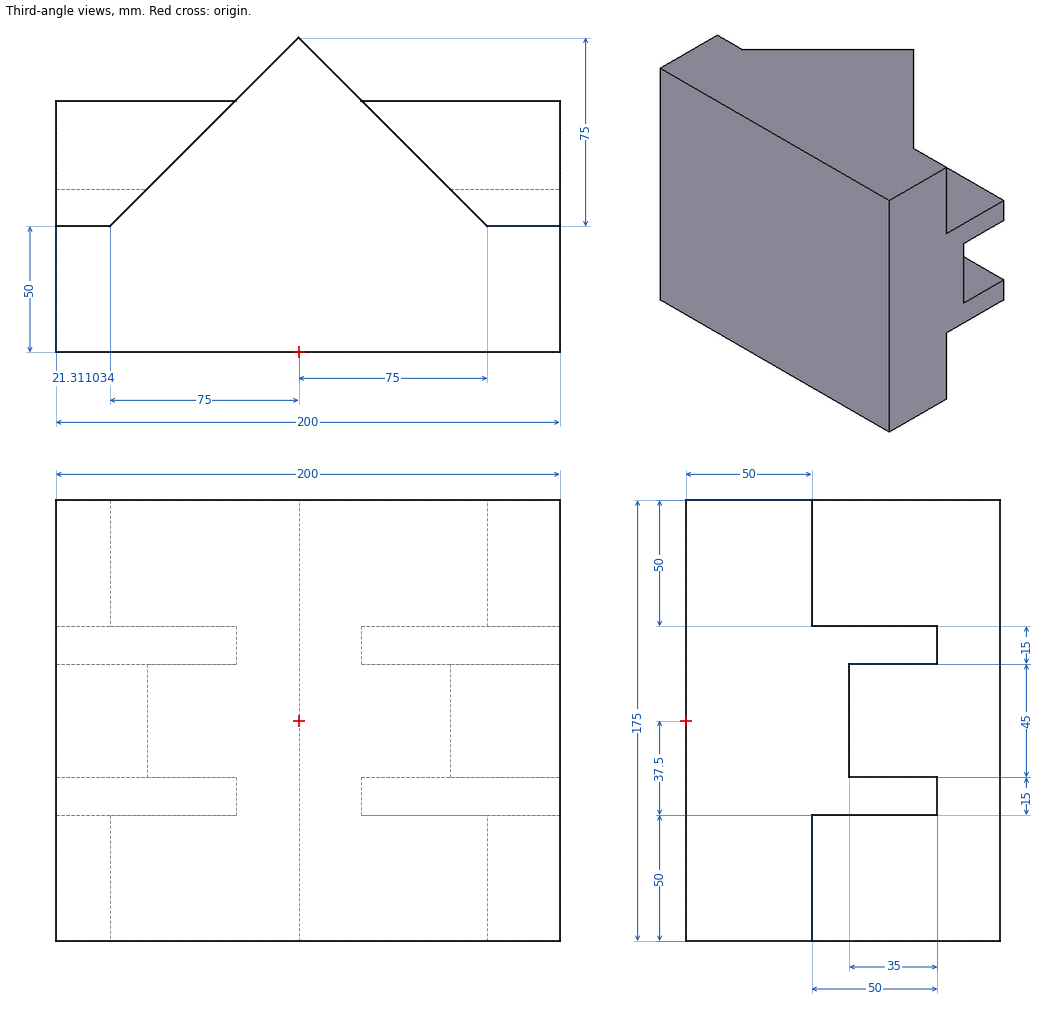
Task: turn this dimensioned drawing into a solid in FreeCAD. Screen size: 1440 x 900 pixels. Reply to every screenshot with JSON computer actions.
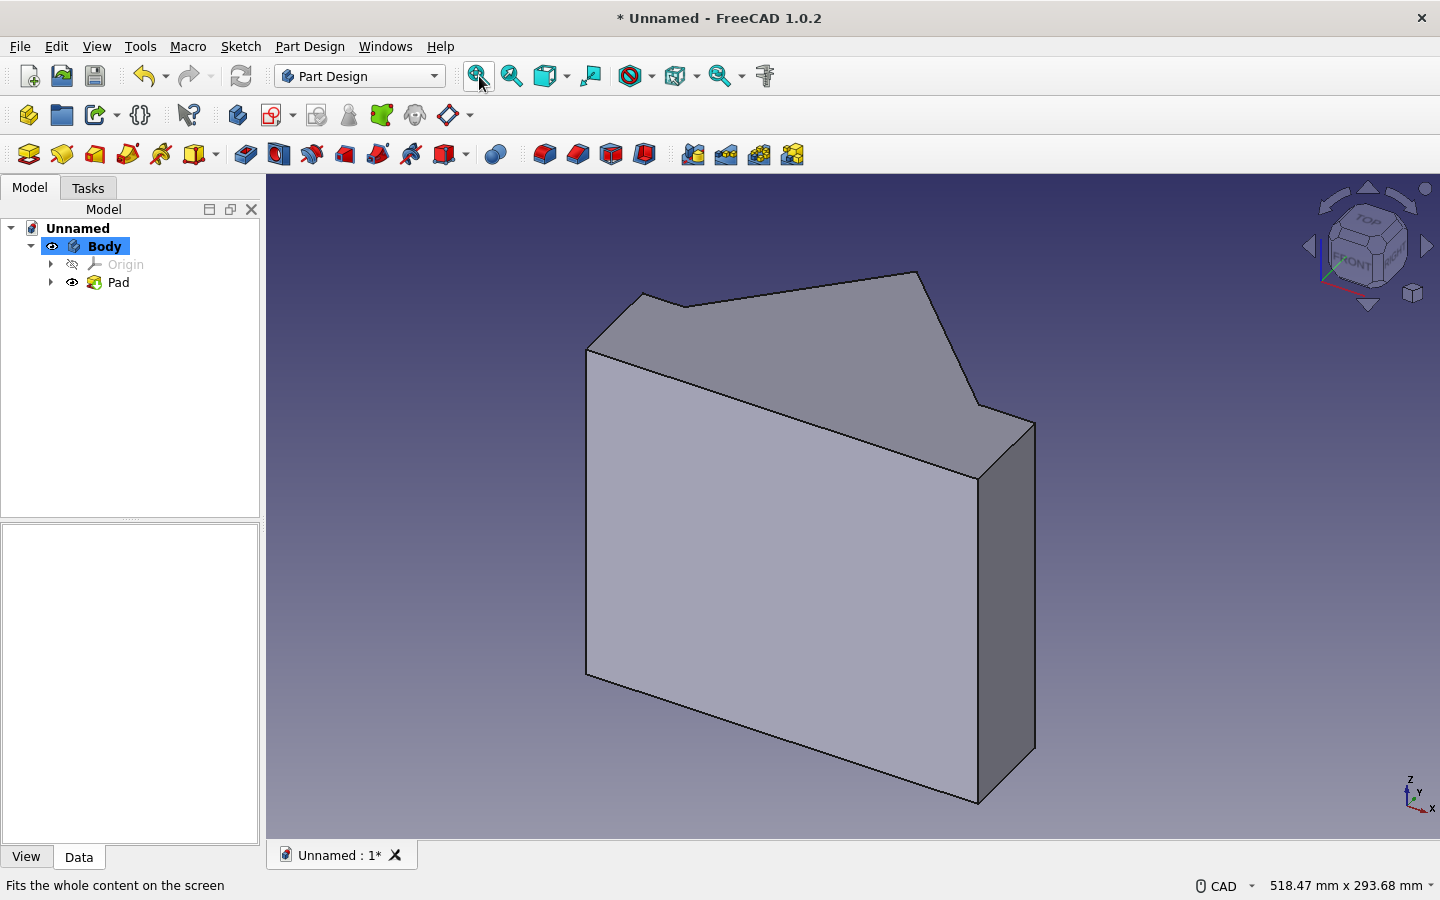
{"action": "key", "text": "6"}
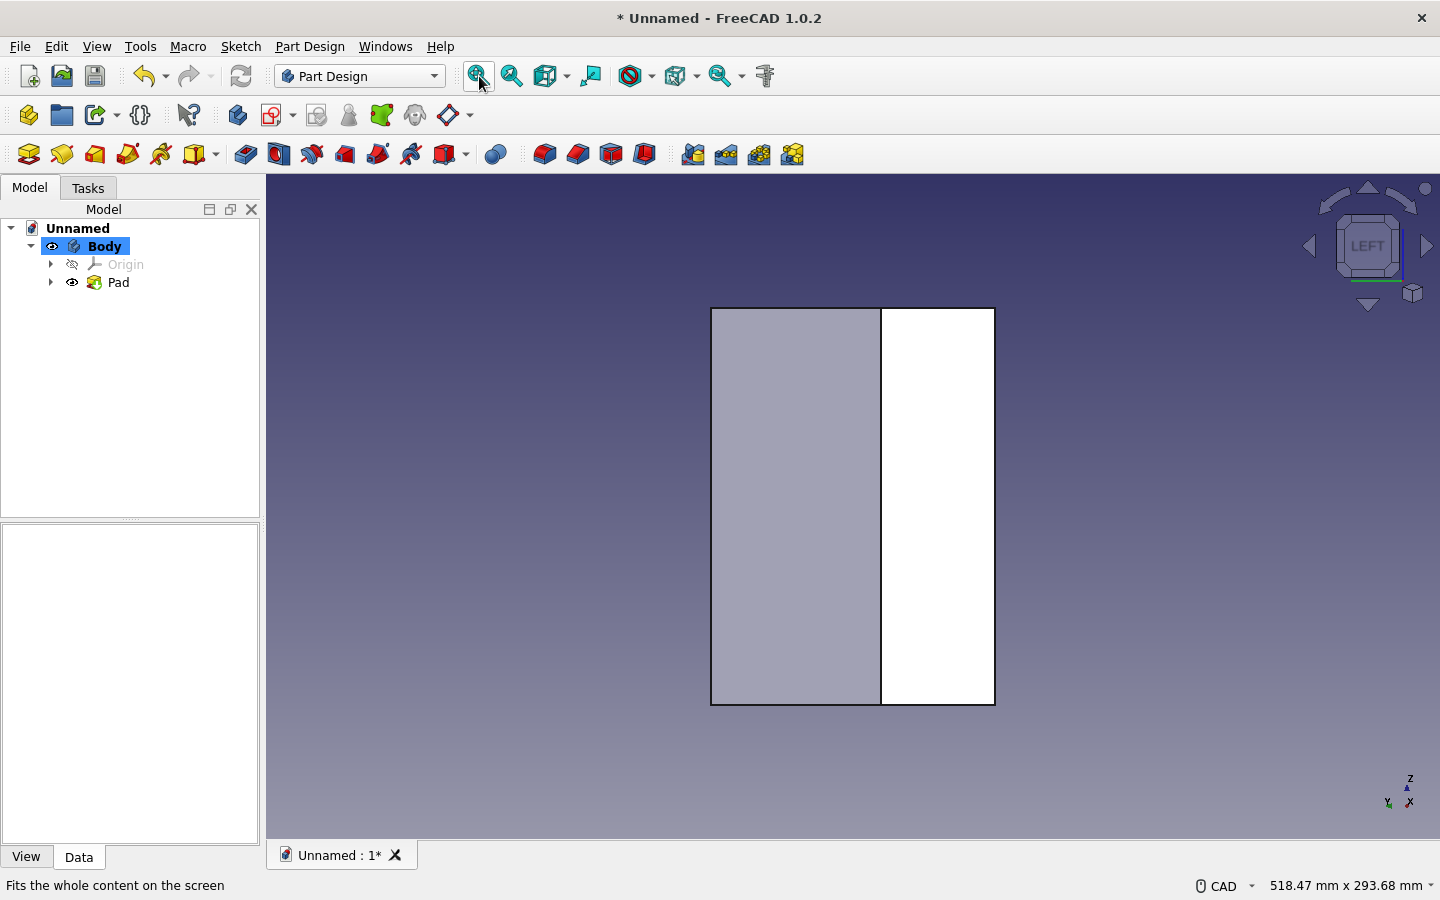
{"action": "left_click", "coordinate": [938, 392]}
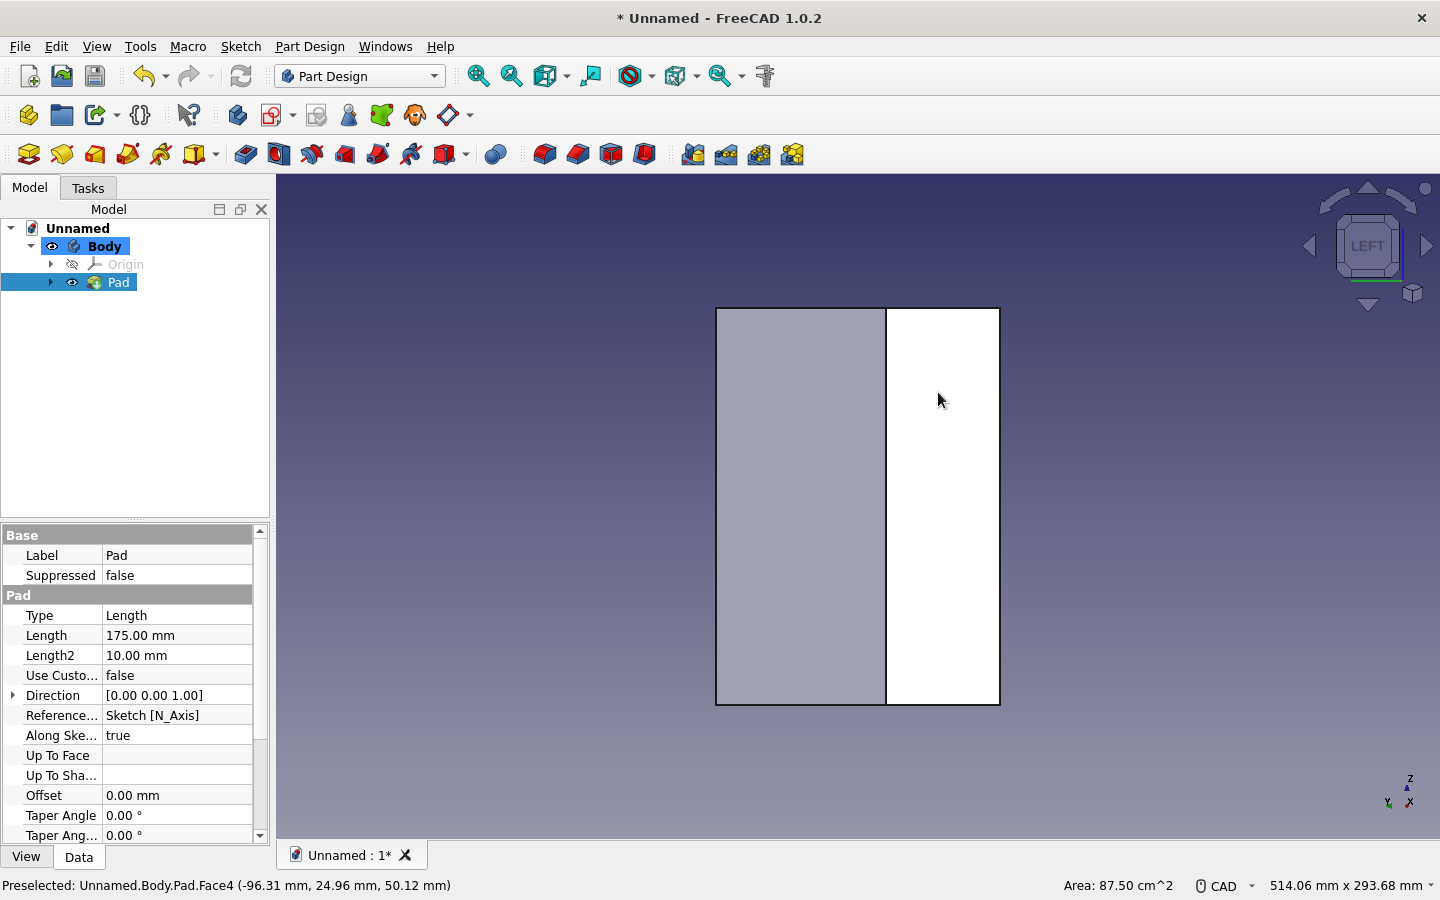
{"action": "left_click", "coordinate": [270, 116]}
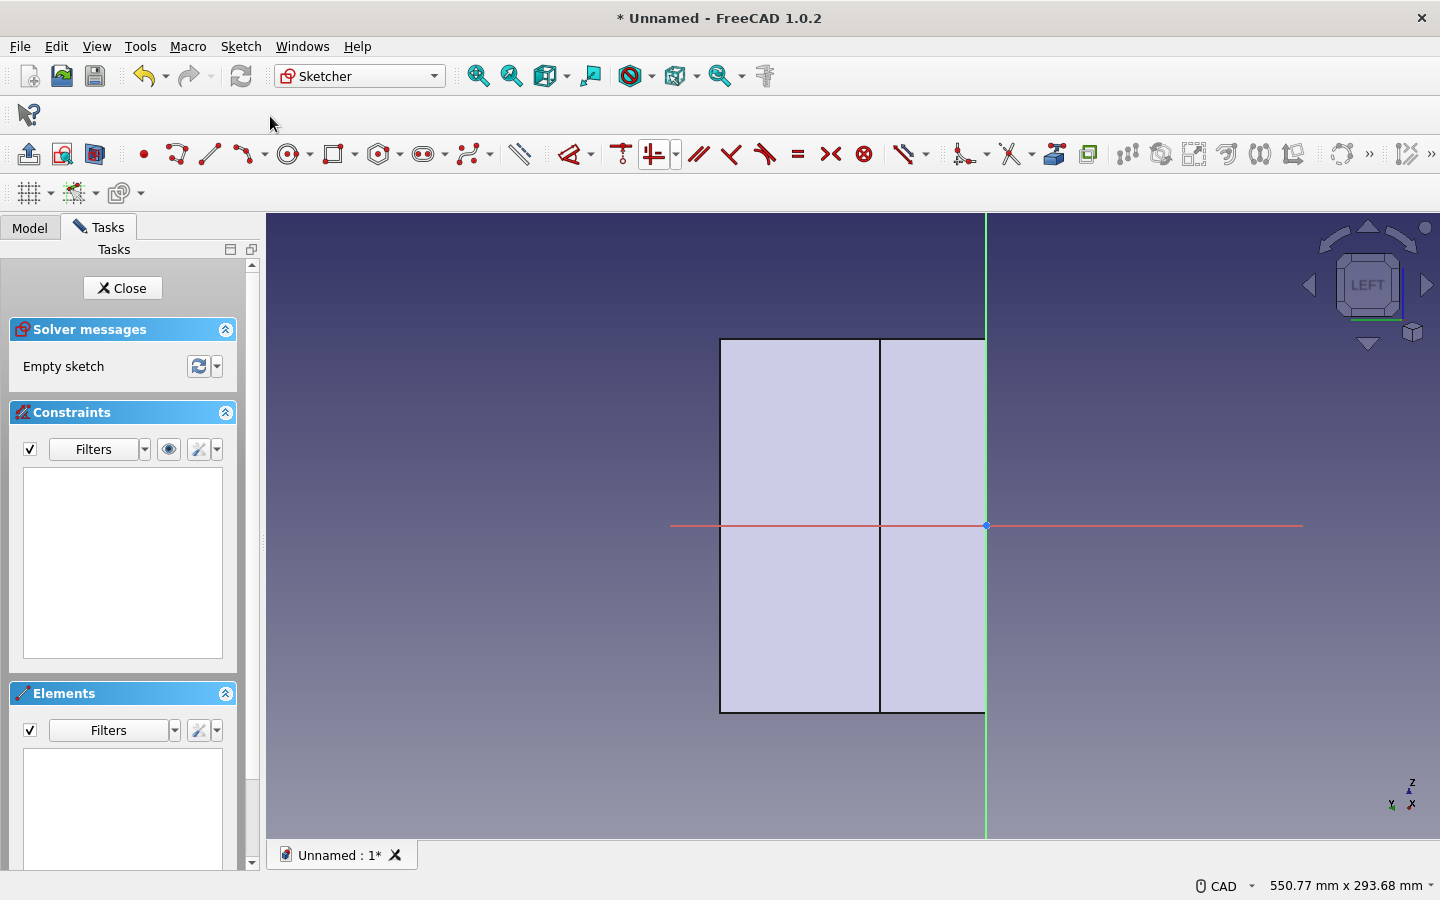
{"action": "left_click", "coordinate": [177, 154]}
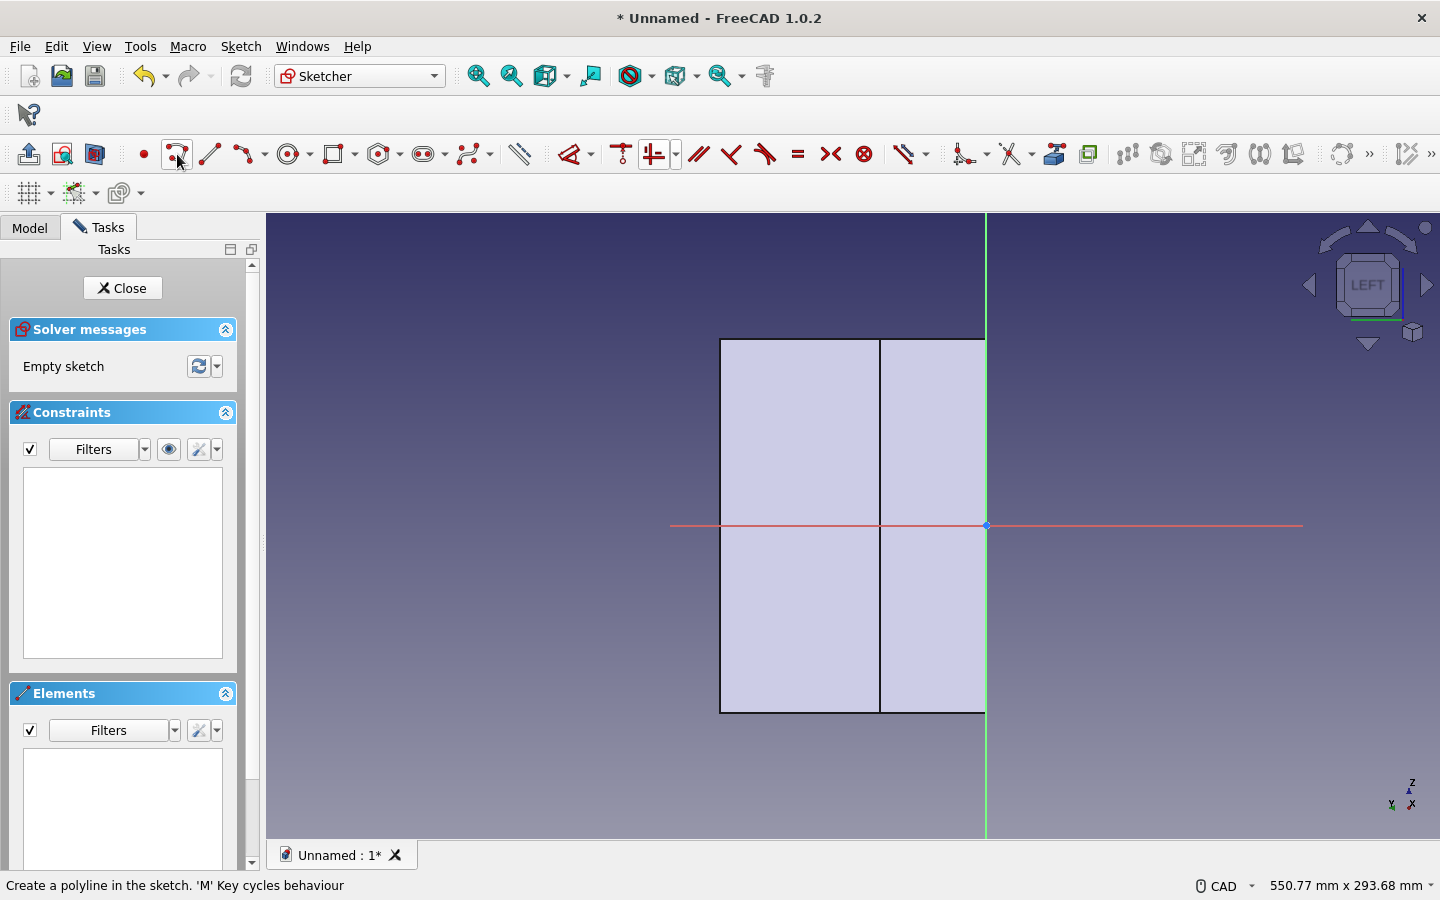
{"action": "left_click", "coordinate": [880, 606]}
{"action": "left_click", "coordinate": [773, 606]}
{"action": "left_click", "coordinate": [773, 574]}
{"action": "left_click", "coordinate": [848, 574]}
{"action": "left_click", "coordinate": [848, 478]}
{"action": "left_click", "coordinate": [773, 478]}
{"action": "left_click", "coordinate": [773, 446]}
{"action": "left_click", "coordinate": [880, 446]}
{"action": "left_click", "coordinate": [880, 339]}
{"action": "left_click", "coordinate": [986, 339]}
{"action": "left_click", "coordinate": [977, 713]}
{"action": "left_click", "coordinate": [880, 713]}
{"action": "left_click", "coordinate": [880, 607]}
{"action": "key", "text": "Escape"}
{"action": "key", "text": "Escape"}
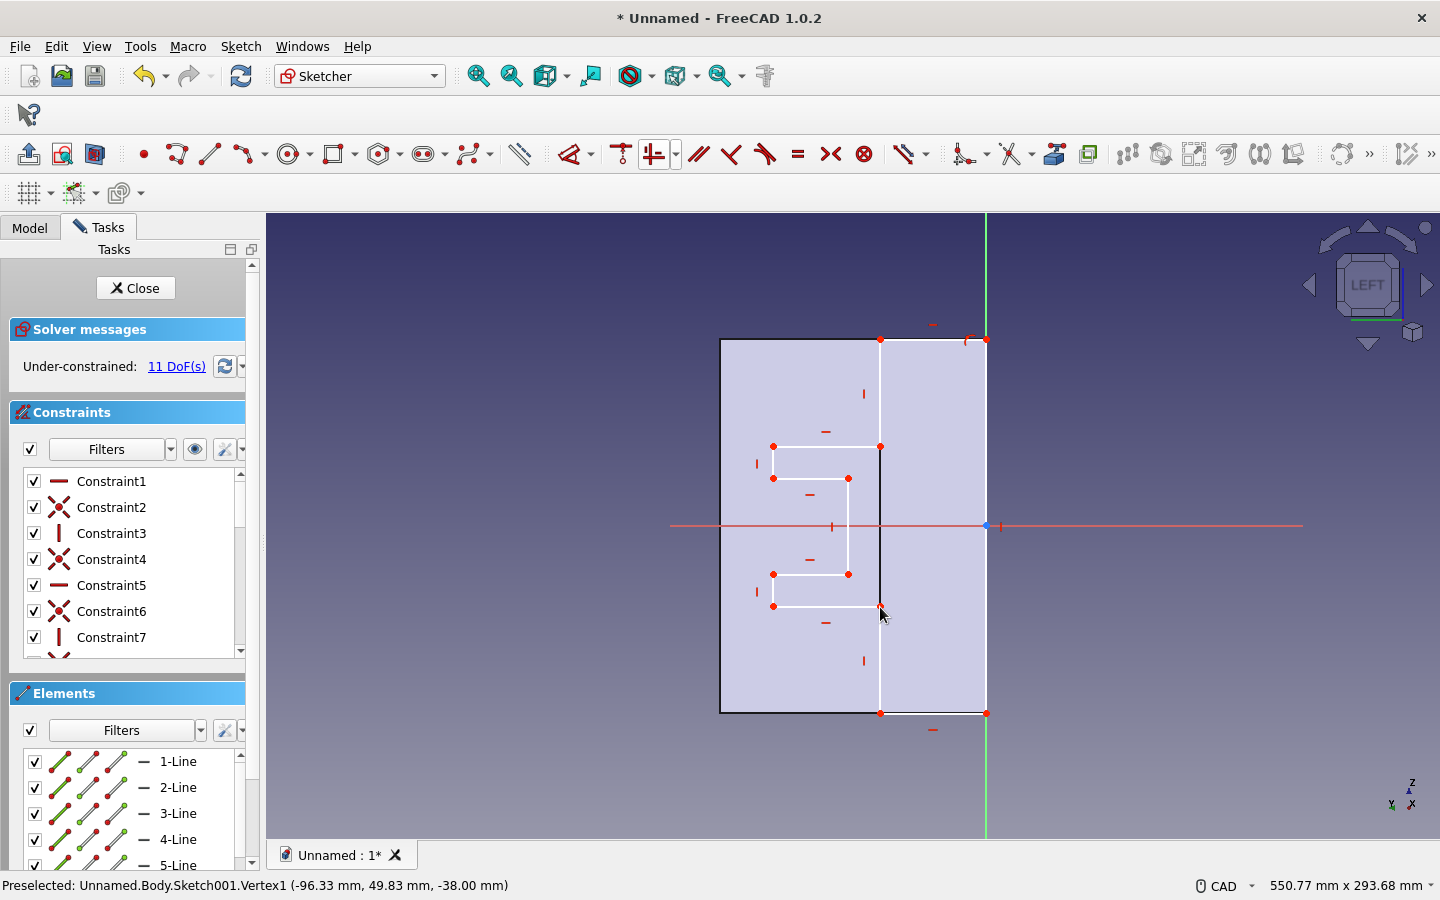
{"action": "left_click", "coordinate": [568, 154]}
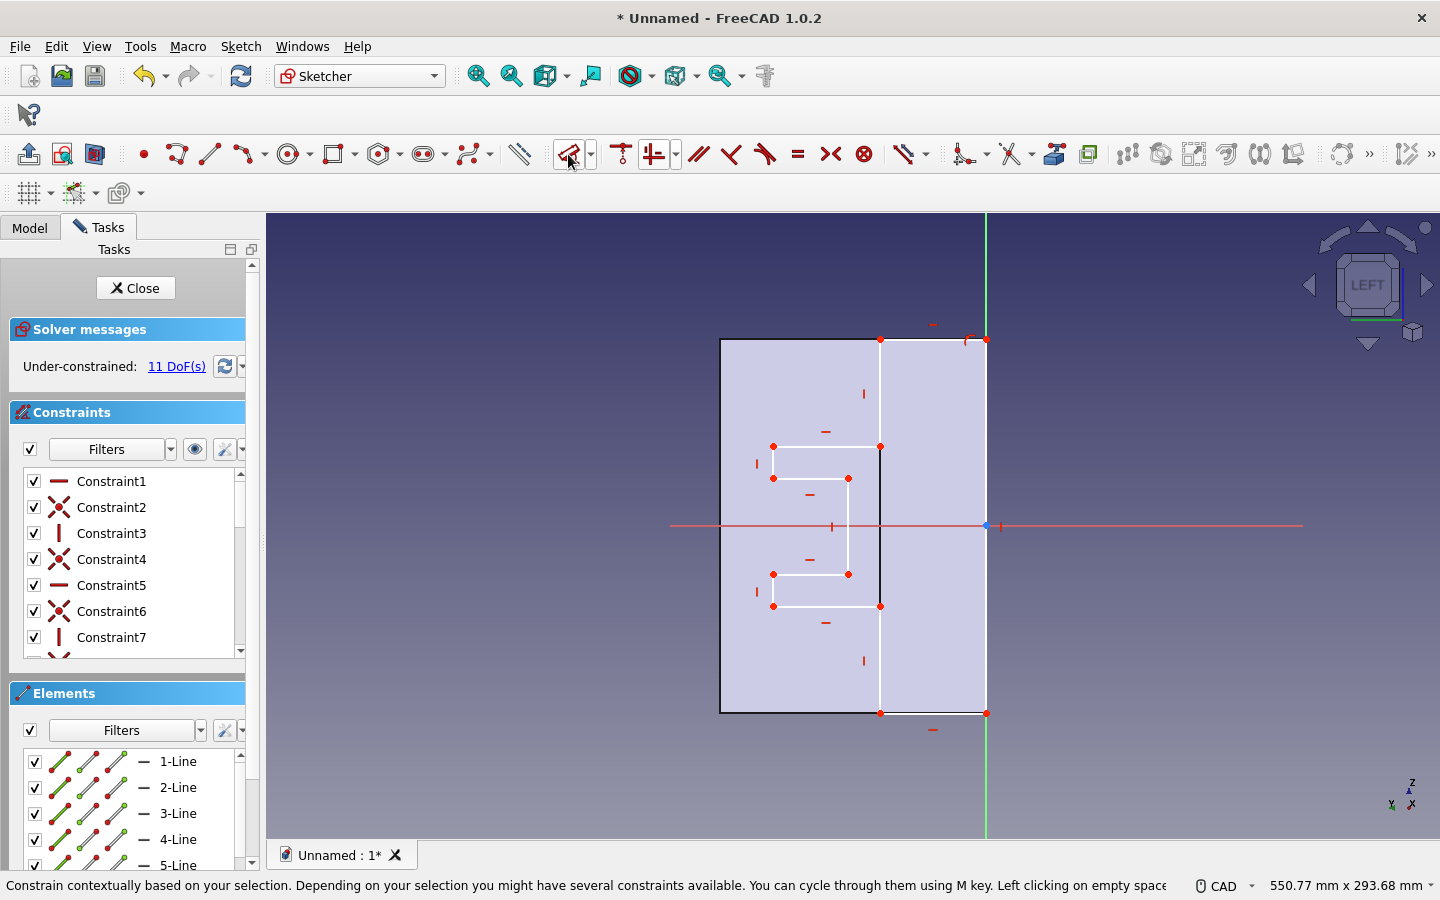
{"action": "left_click", "coordinate": [848, 607]}
{"action": "left_click", "coordinate": [826, 641]}